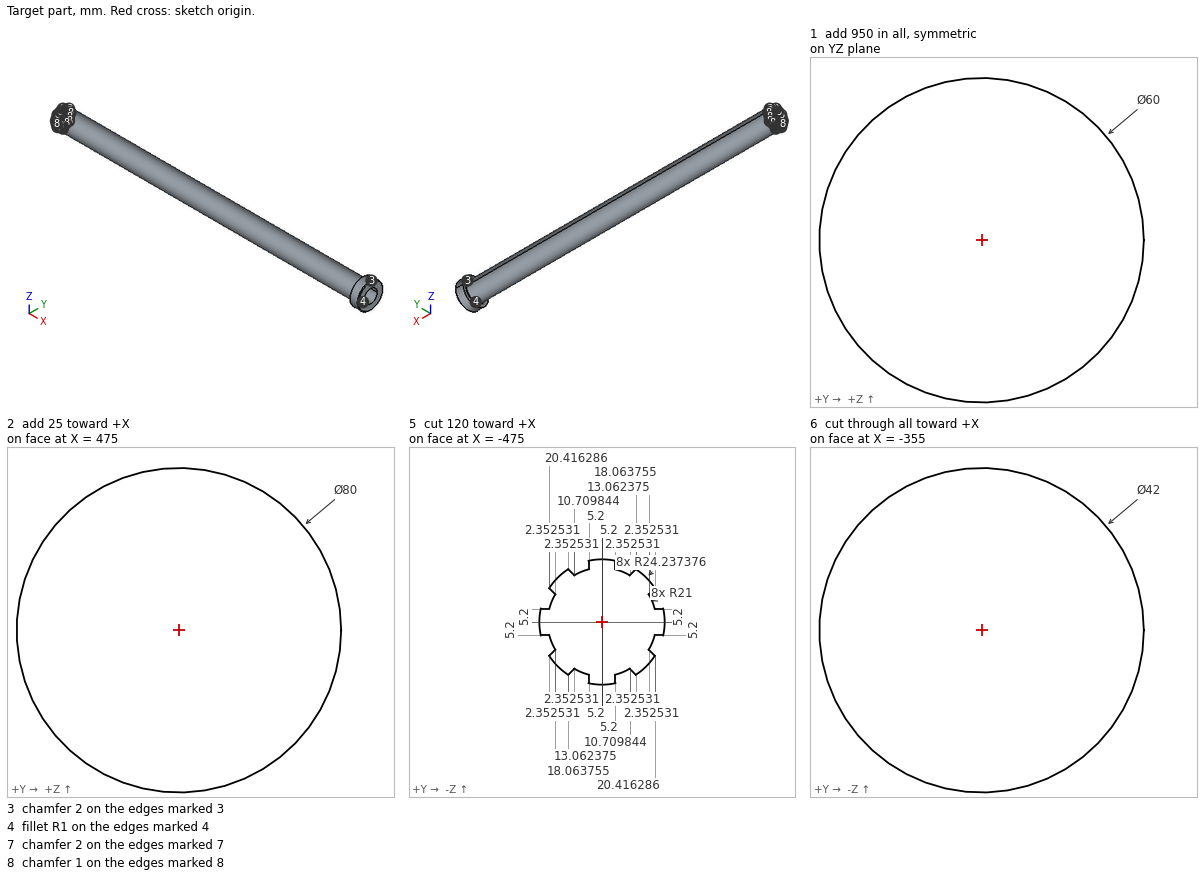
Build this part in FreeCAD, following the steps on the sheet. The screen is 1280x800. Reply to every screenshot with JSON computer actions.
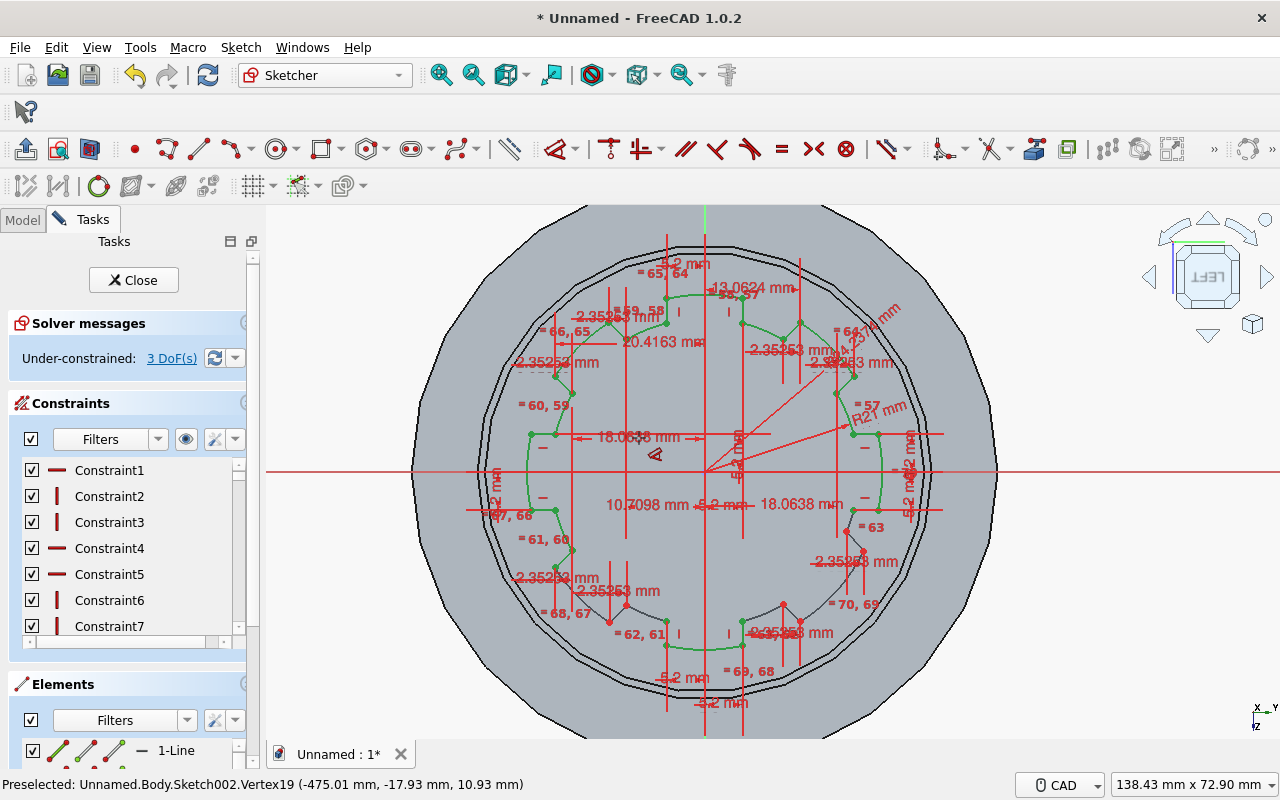
{"action": "left_click", "coordinate": [610, 622]}
{"action": "left_click", "coordinate": [657, 656]}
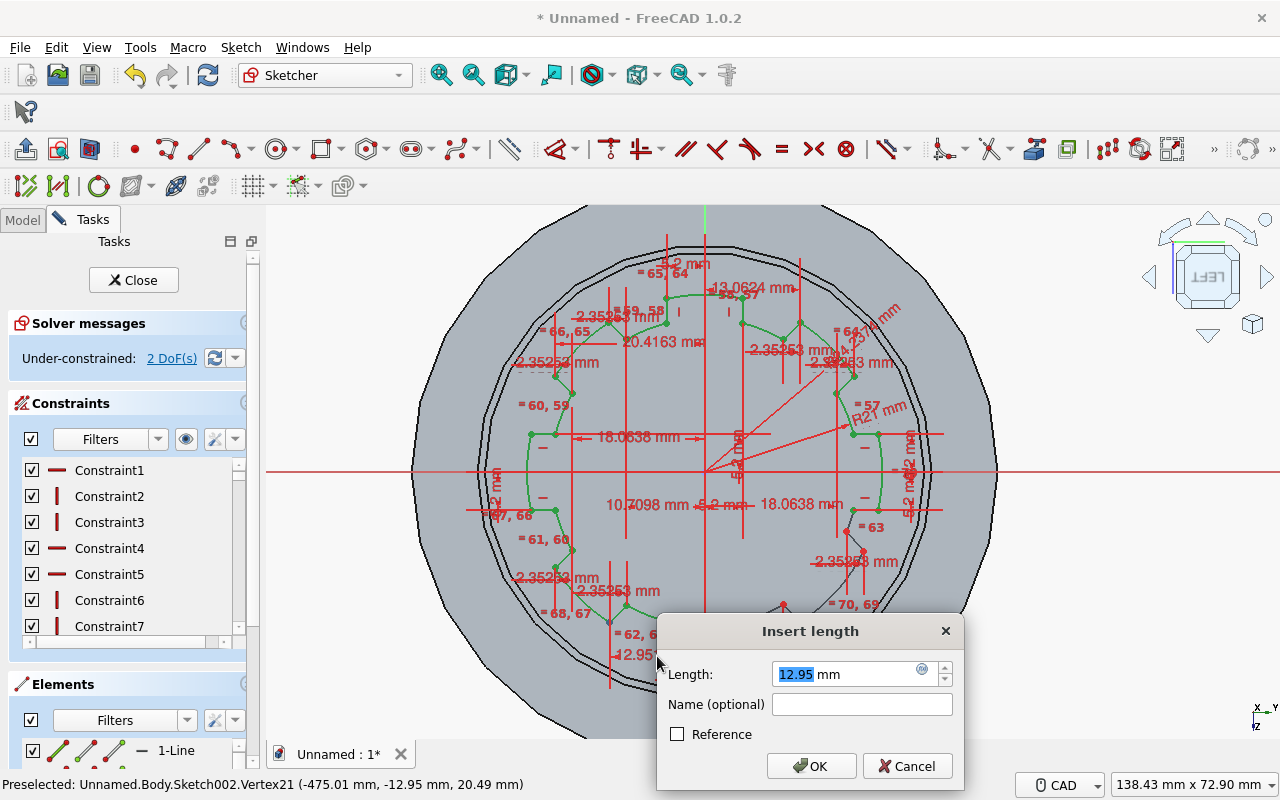
{"action": "type", "text": "13.062375"}
{"action": "key", "text": "Return"}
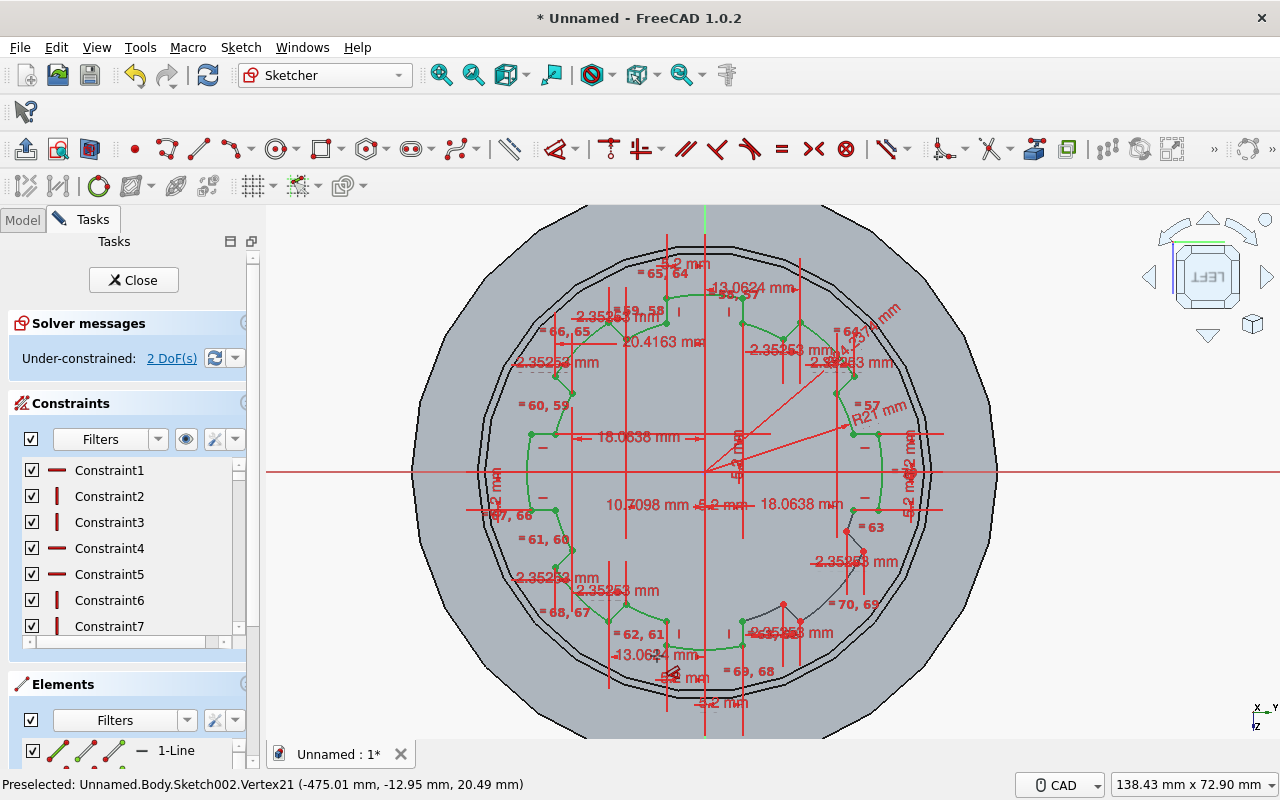
{"action": "left_click", "coordinate": [783, 605]}
{"action": "left_click", "coordinate": [762, 663]}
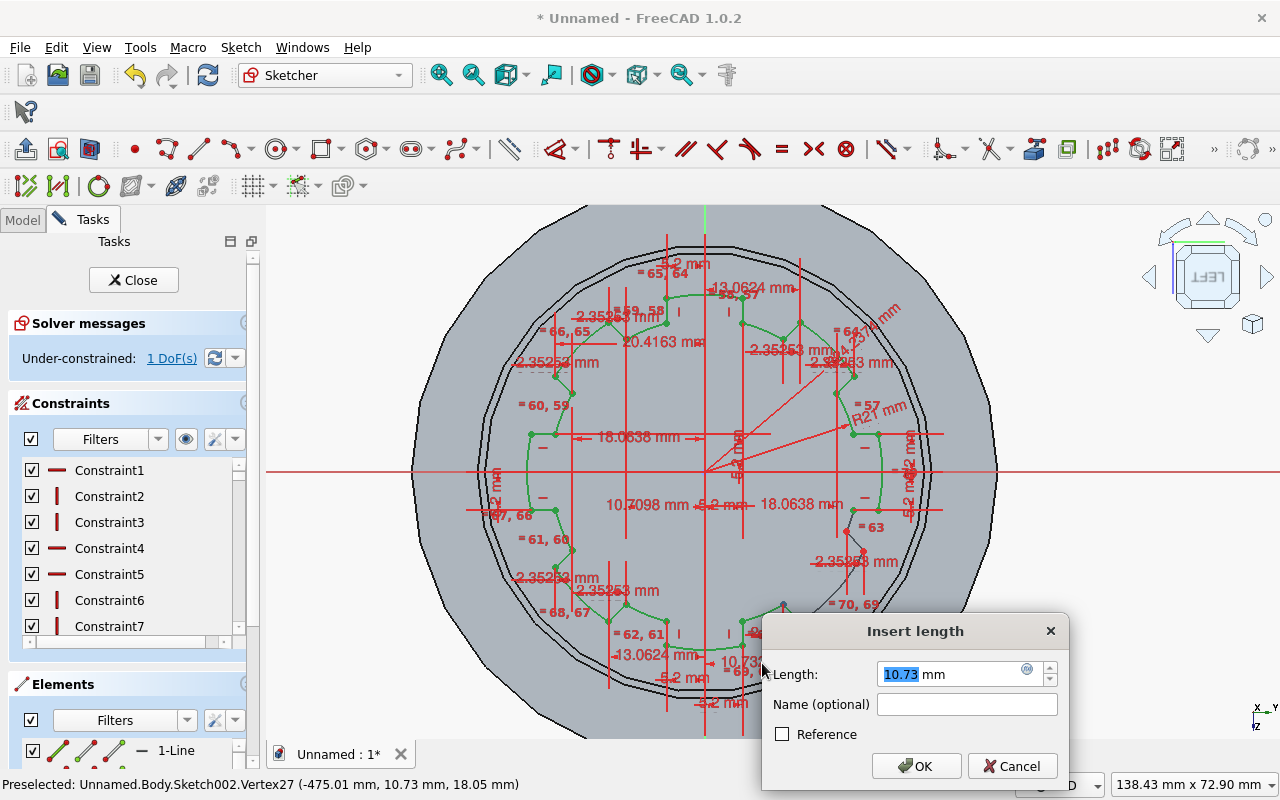
{"action": "type", "text": "10.709844"}
{"action": "key", "text": "Return"}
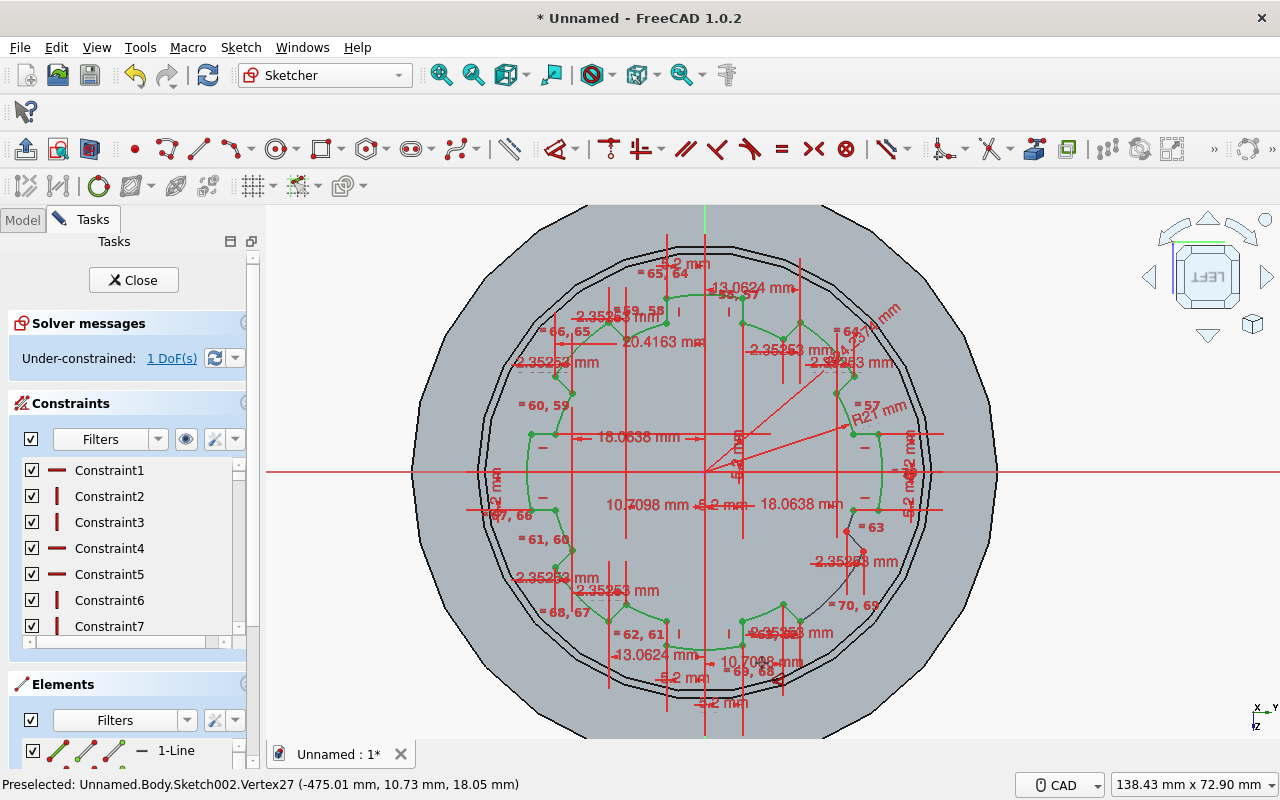
{"action": "left_click", "coordinate": [864, 551]}
{"action": "left_click", "coordinate": [748, 585]}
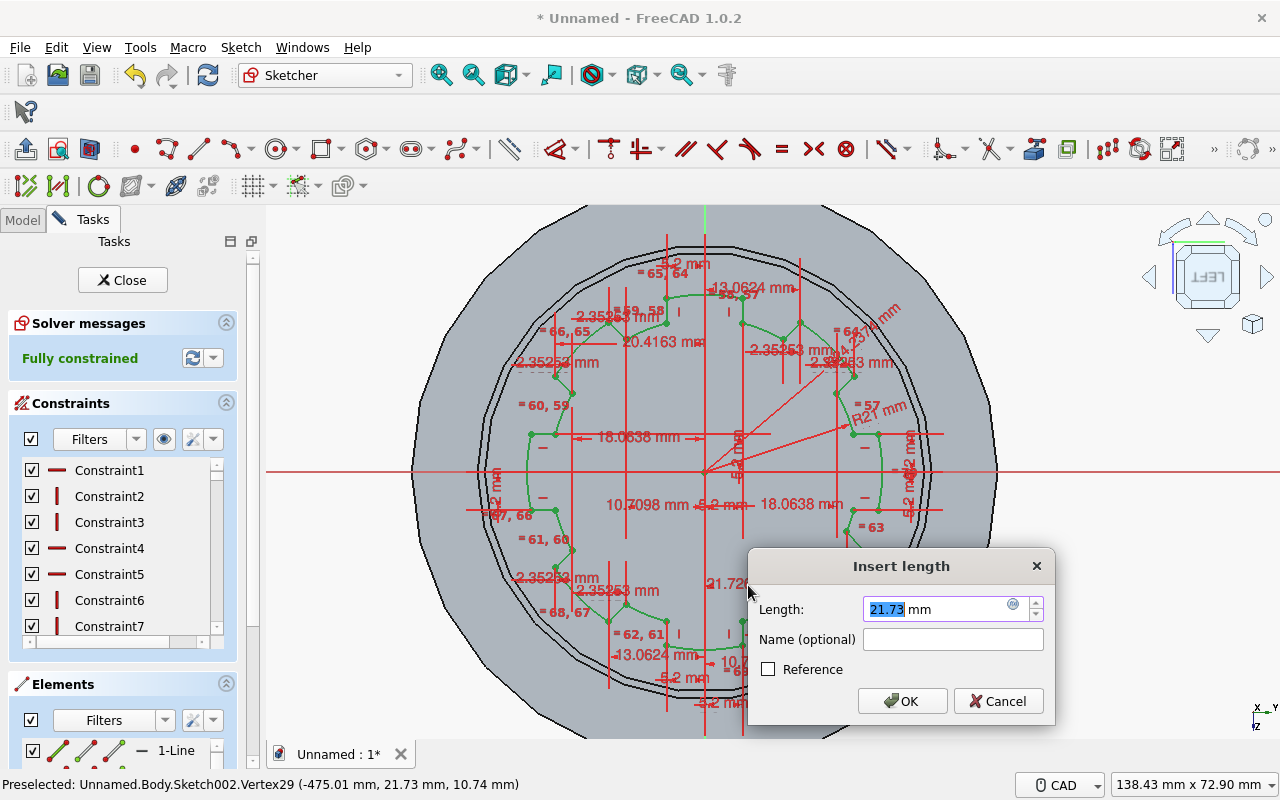
{"action": "type", "text": "20.416286"}
{"action": "key", "text": "Return"}
{"action": "key", "text": "Escape"}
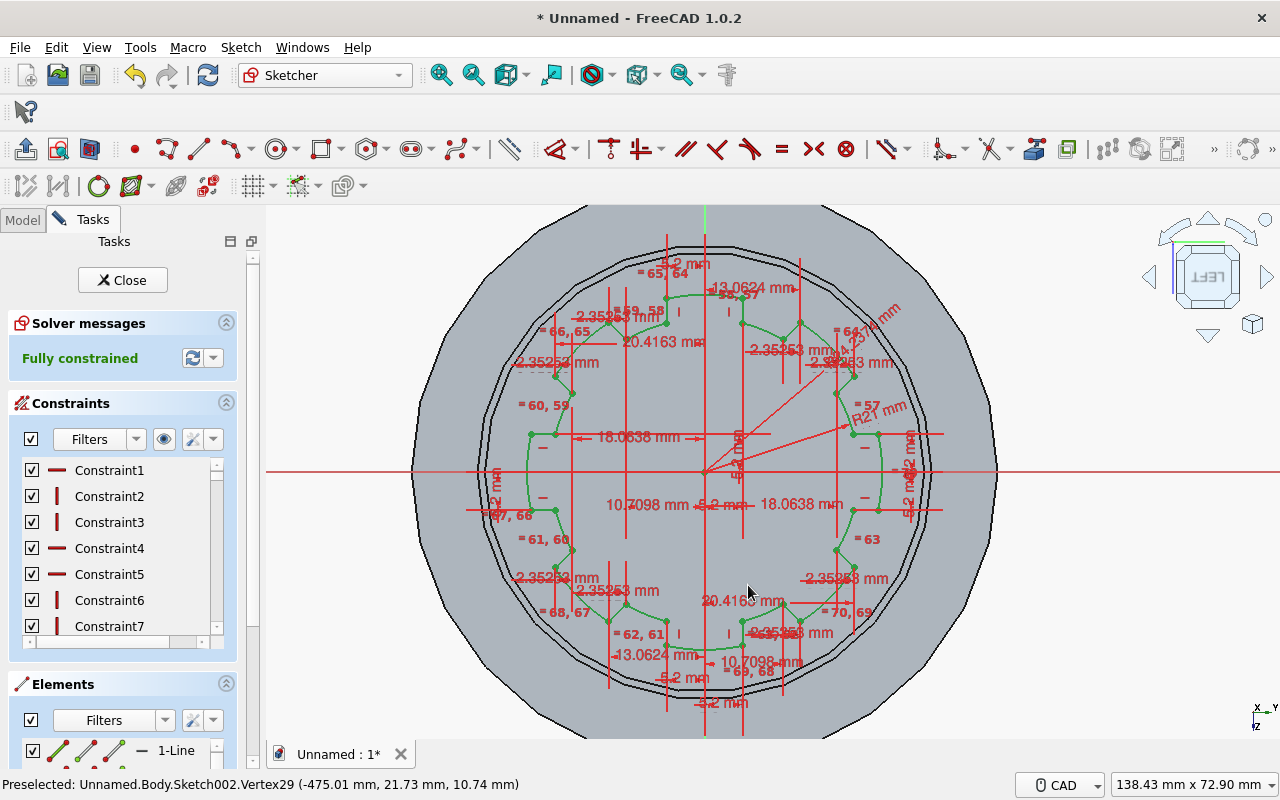
{"action": "left_click", "coordinate": [123, 280]}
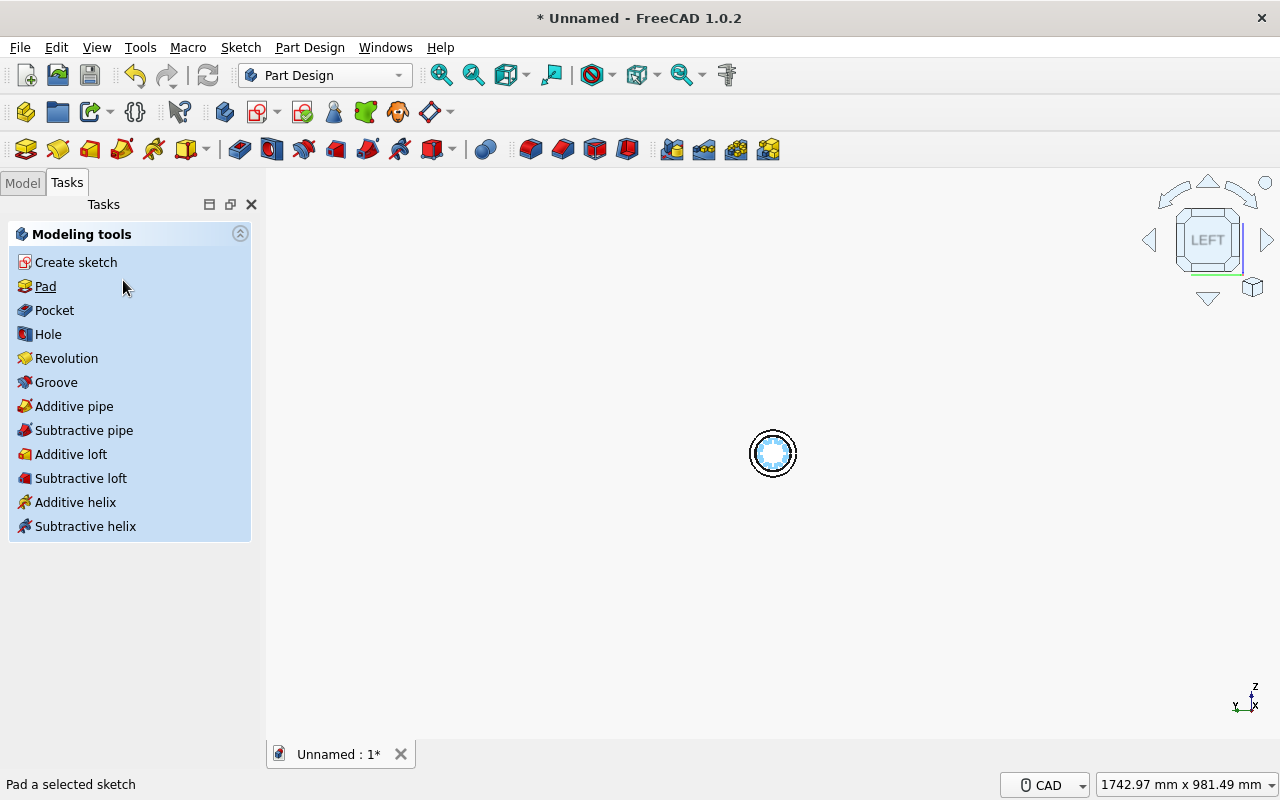
{"action": "left_click", "coordinate": [240, 150]}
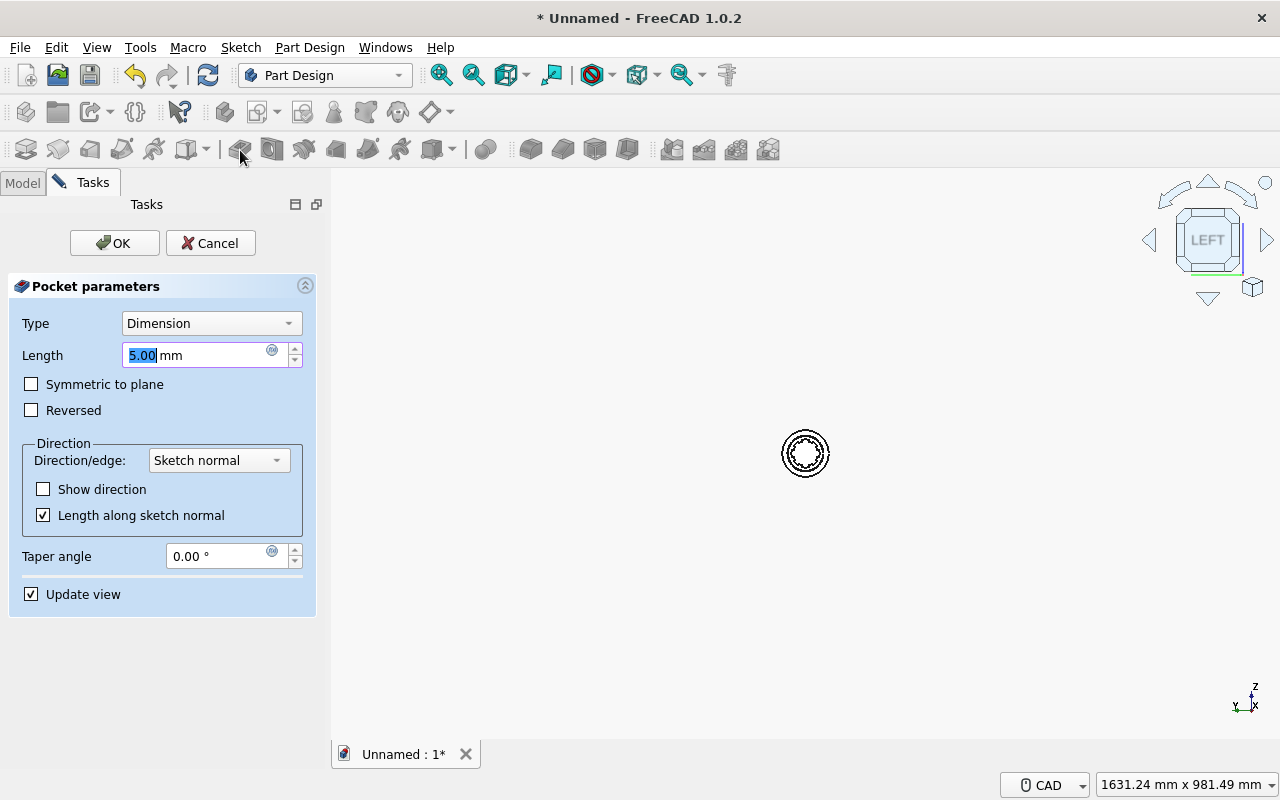
{"action": "type", "text": "120"}
{"action": "key", "text": "Tab"}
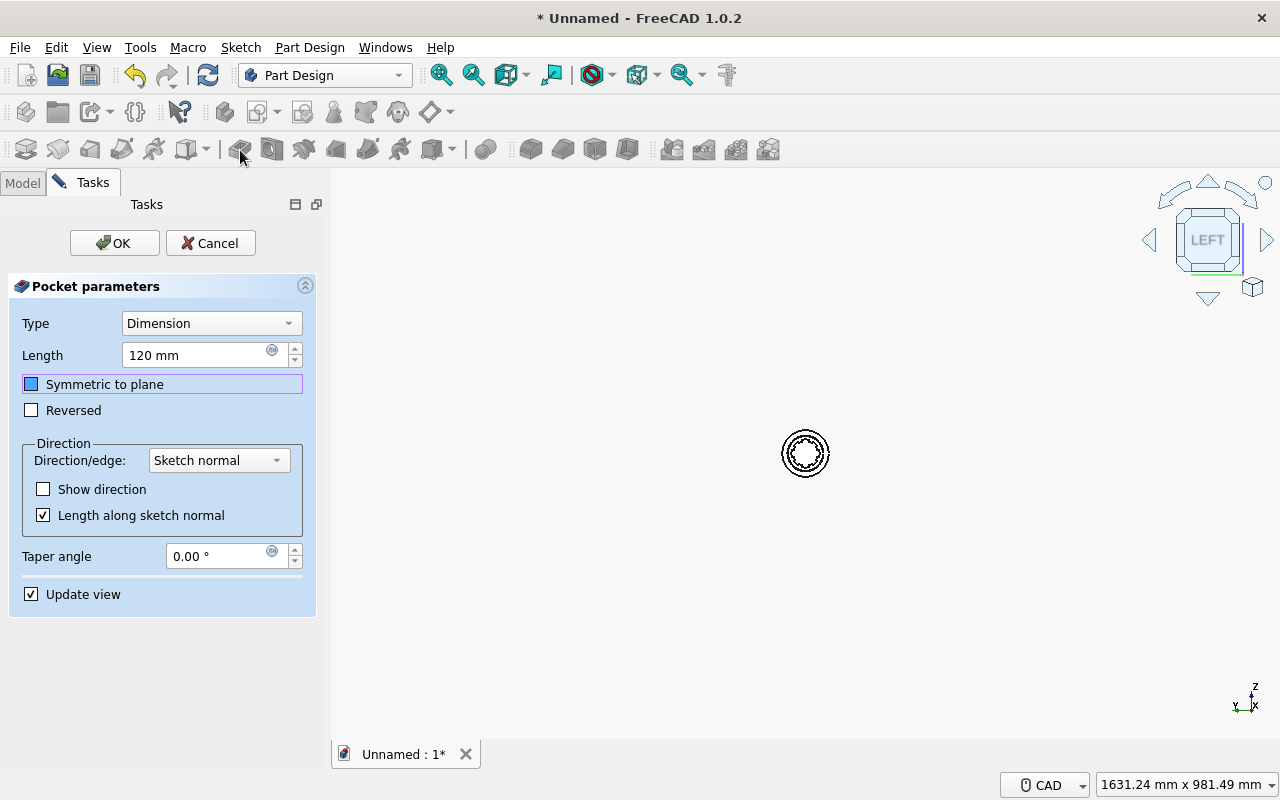
{"action": "left_click", "coordinate": [115, 243]}